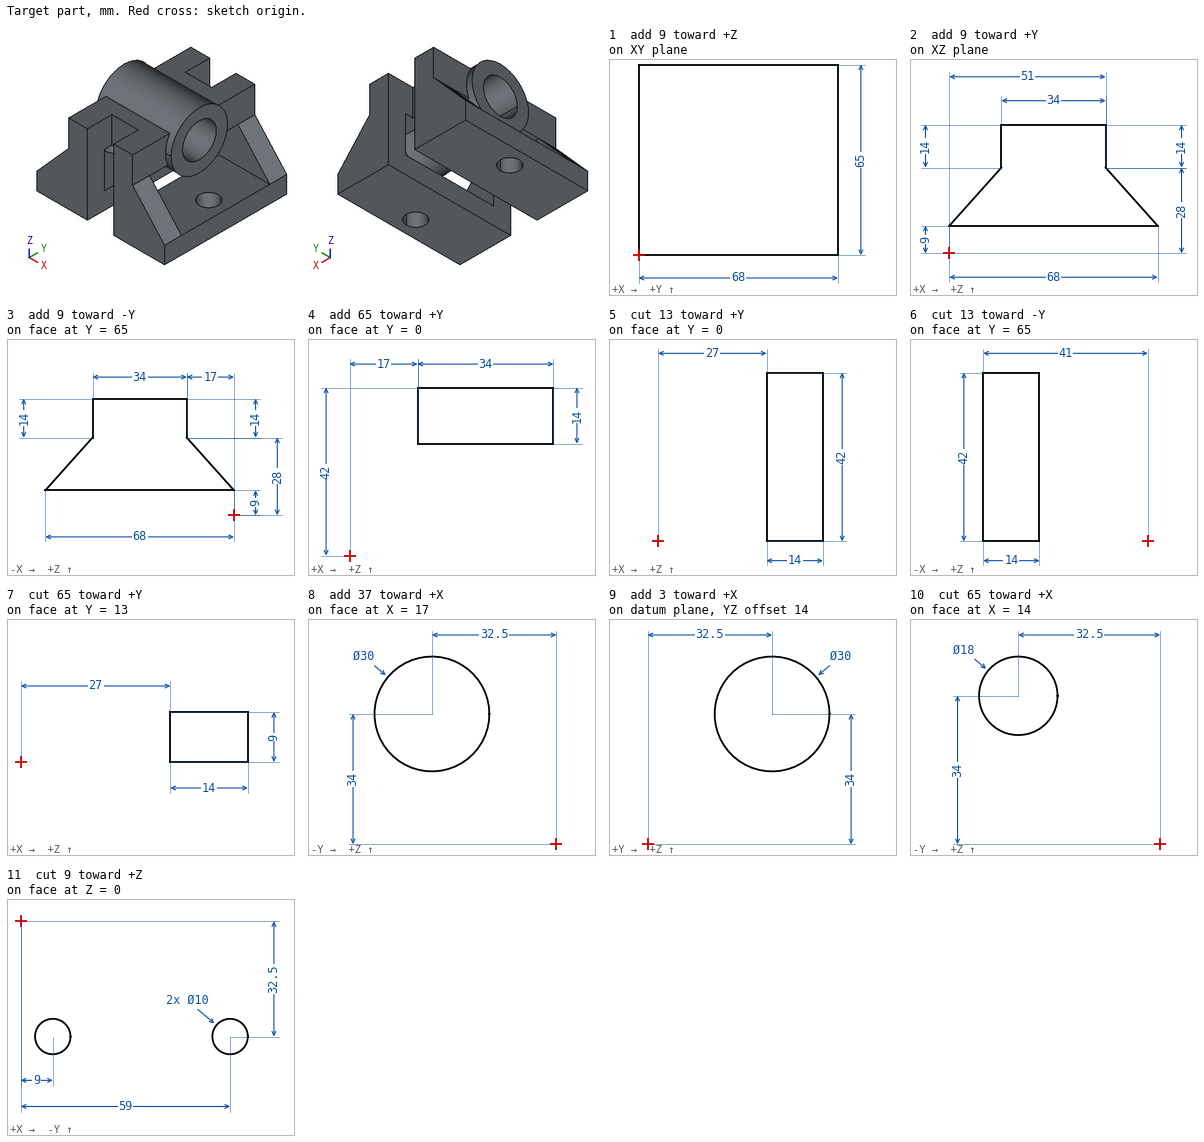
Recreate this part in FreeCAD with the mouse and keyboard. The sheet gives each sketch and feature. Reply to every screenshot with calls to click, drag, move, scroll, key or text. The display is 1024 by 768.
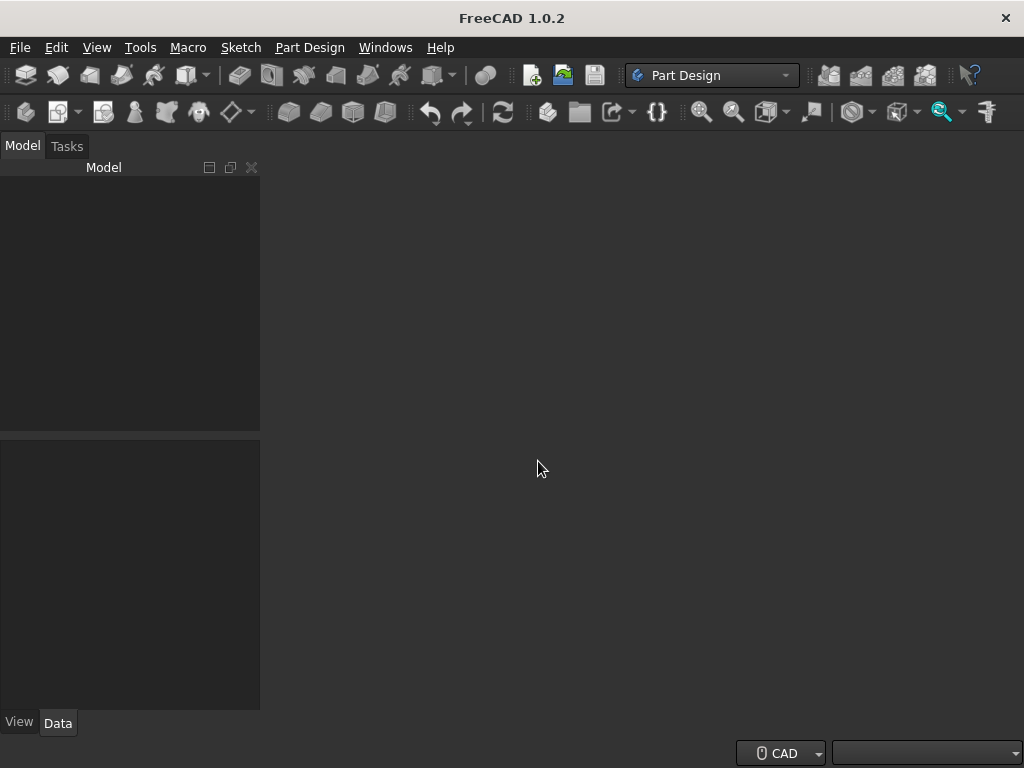
click(532, 76)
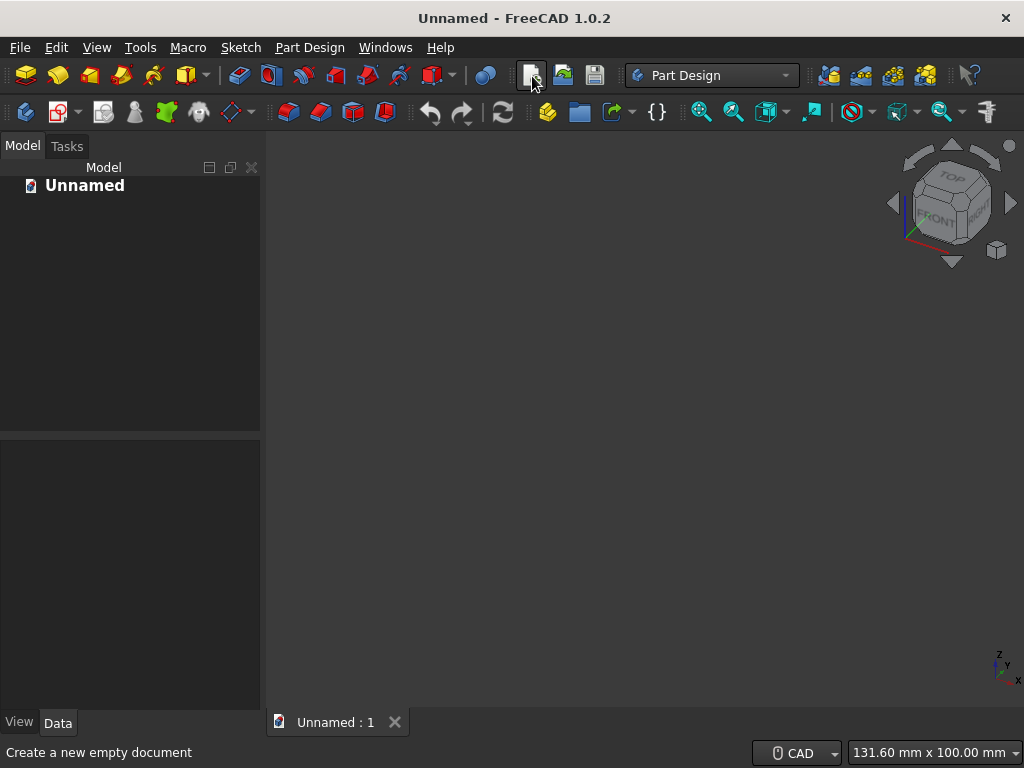
click(58, 112)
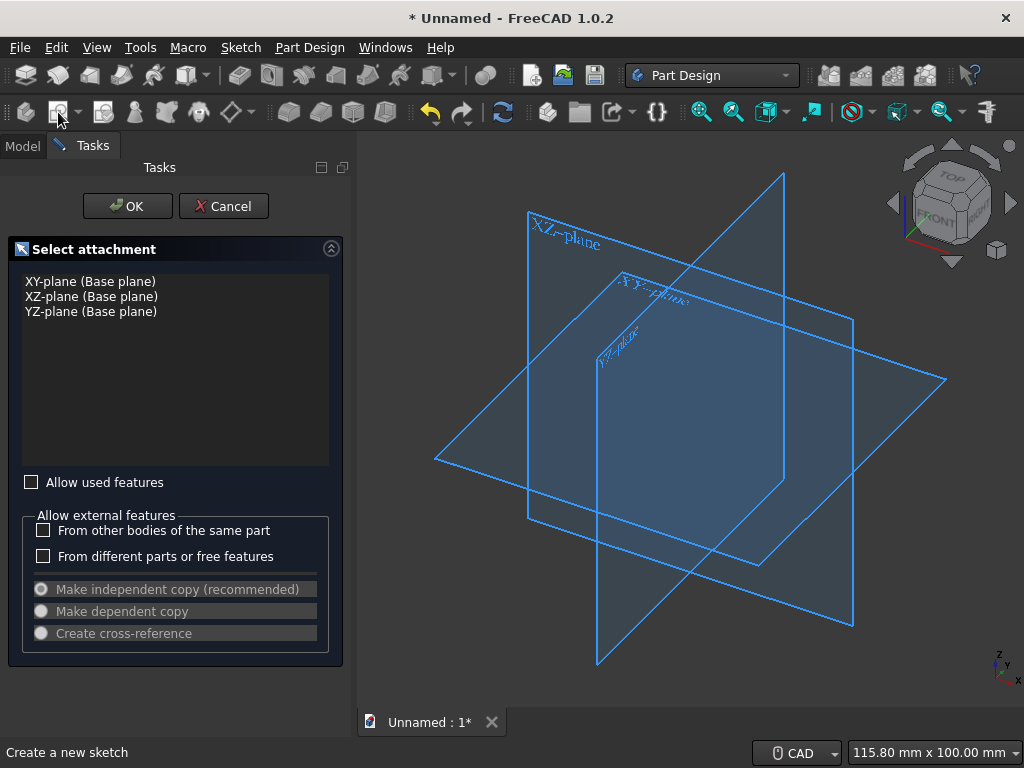
click(82, 282)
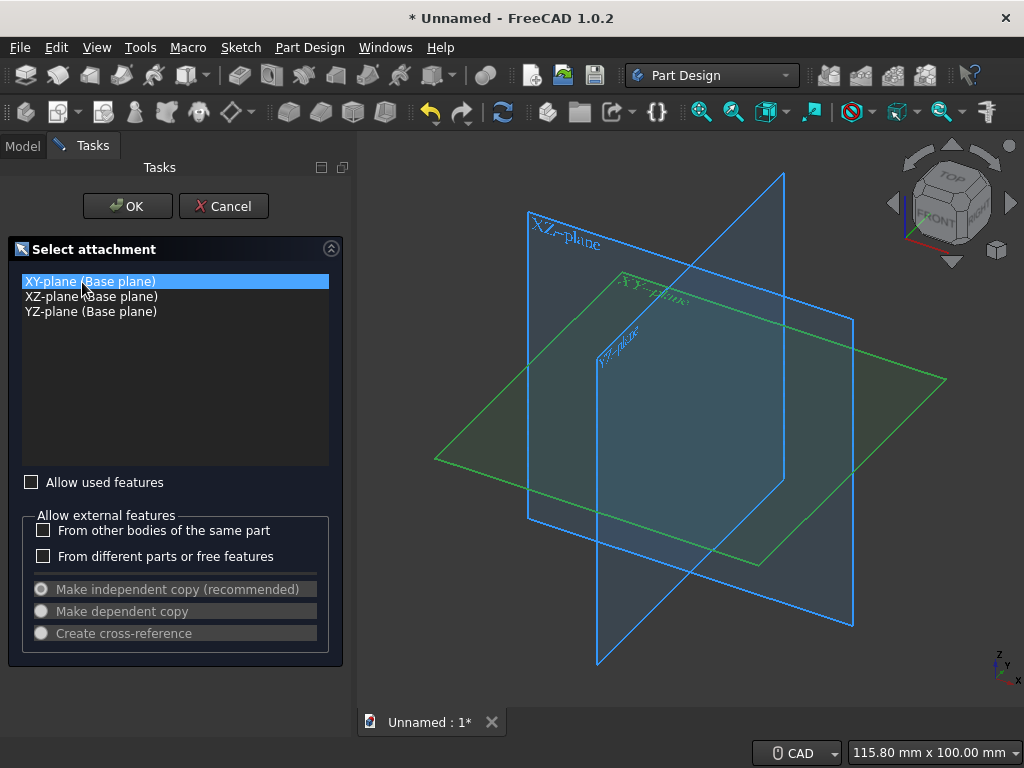
click(128, 206)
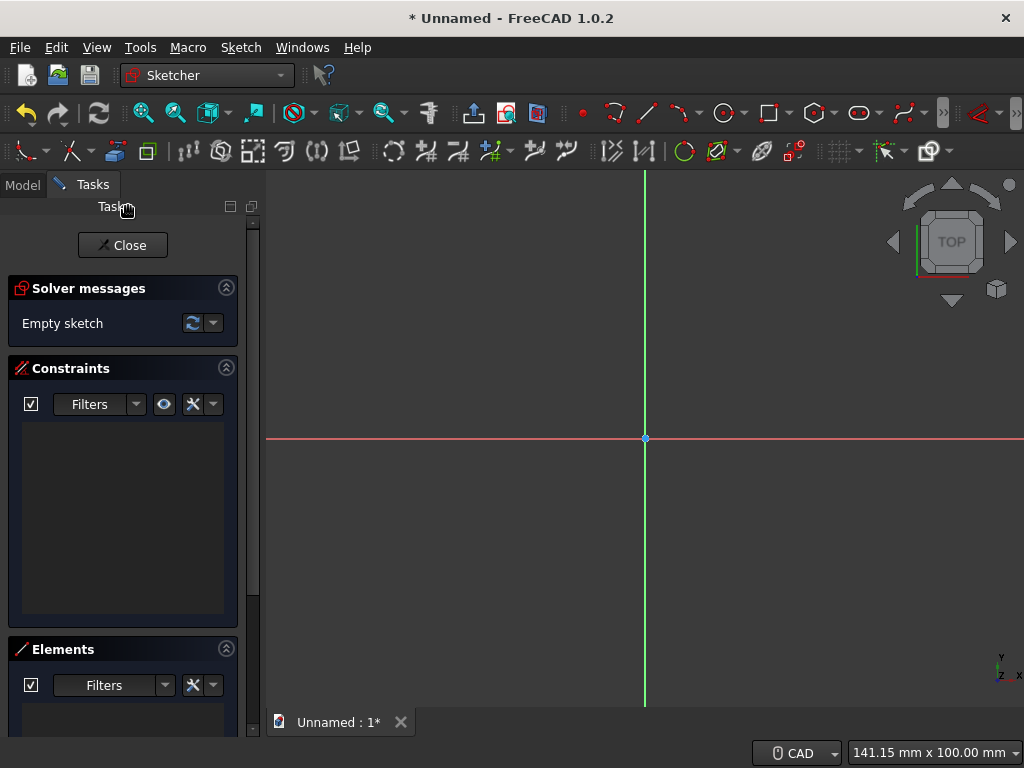
scroll(294, 679, down, 2)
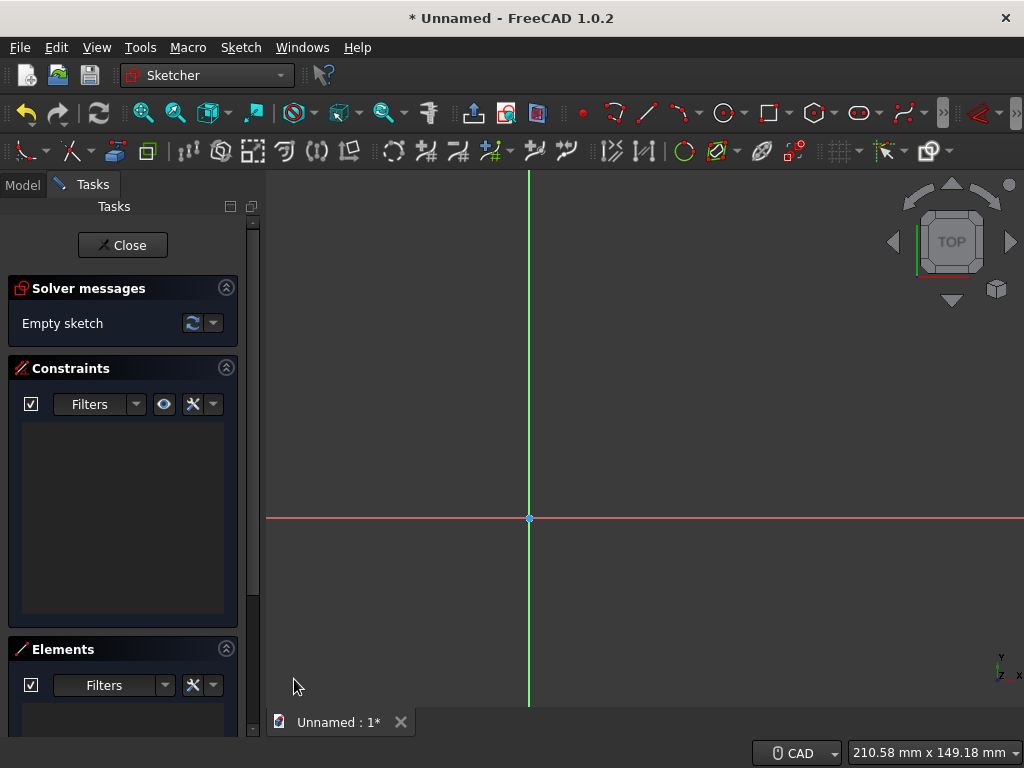
scroll(805, 325, up, 2)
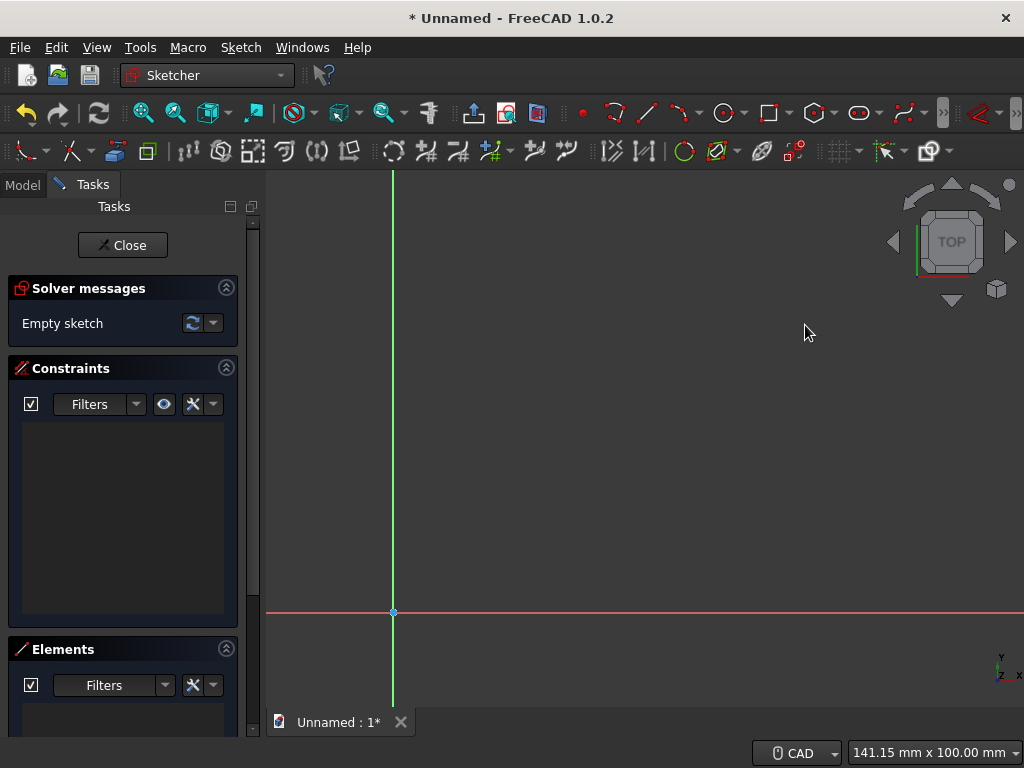
key(g)
key(r)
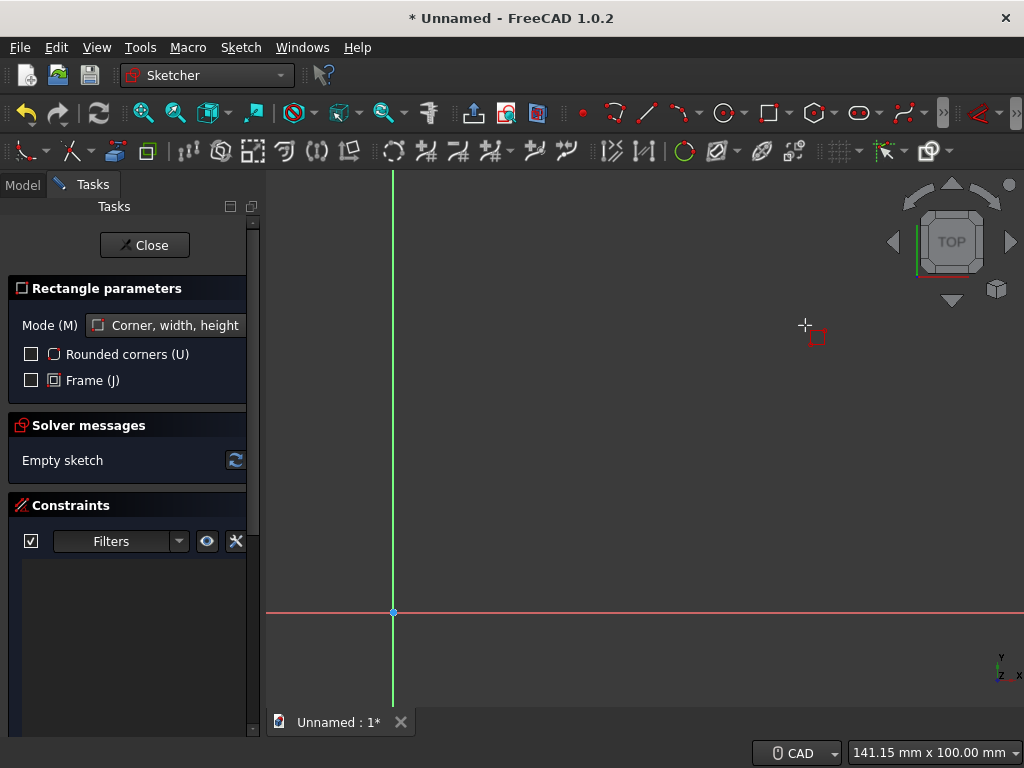
click(393, 613)
move(759, 264)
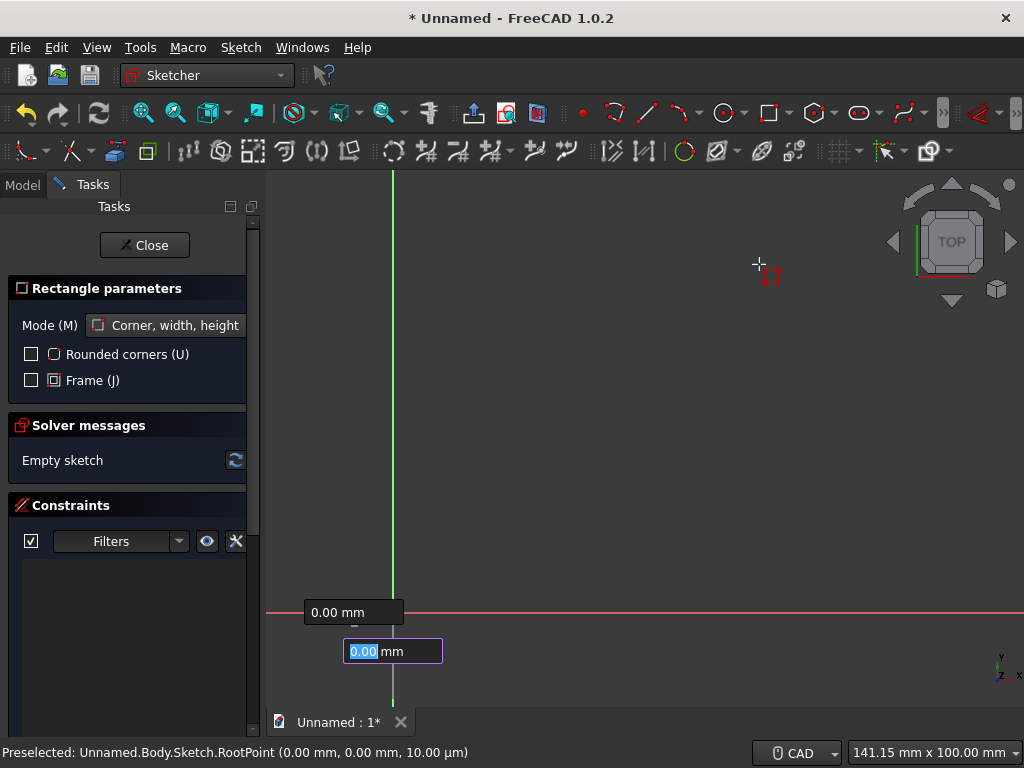
text(68)
key(Tab)
text(65)
key(Return)
key(Escape)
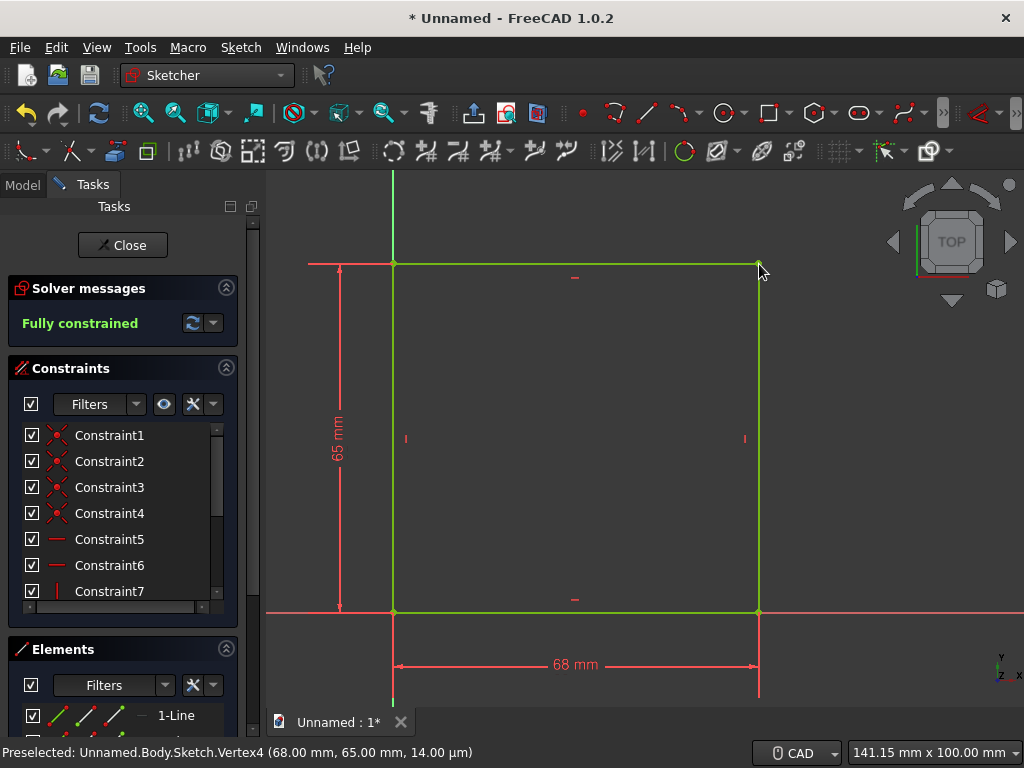
click(123, 245)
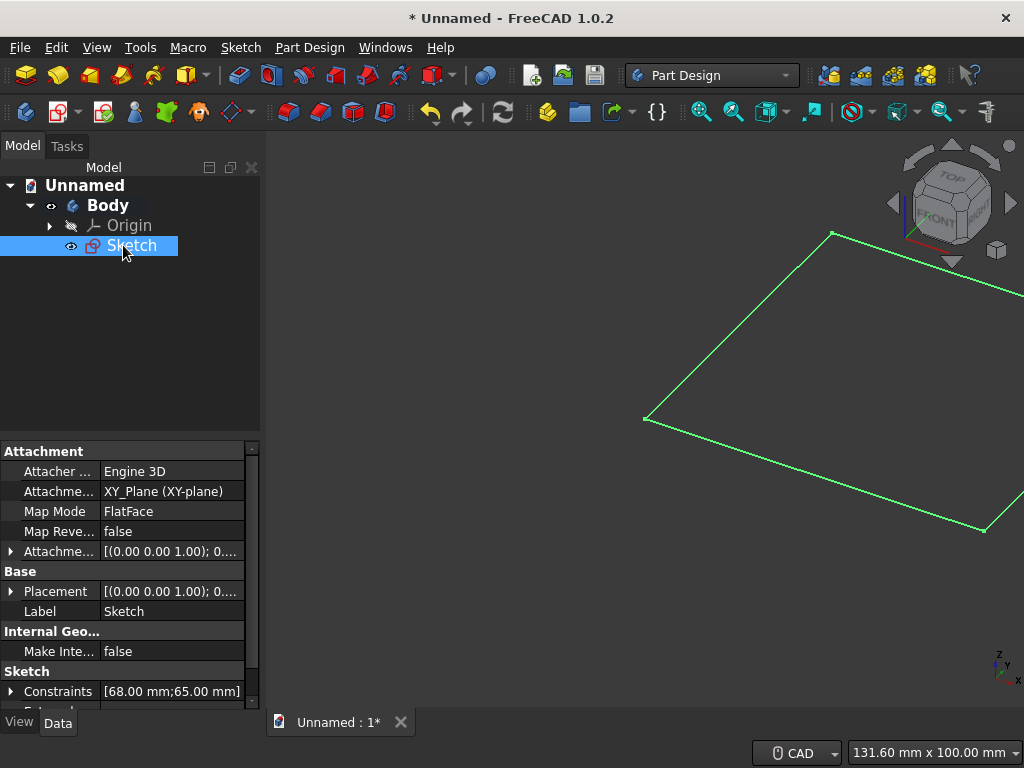
click(26, 76)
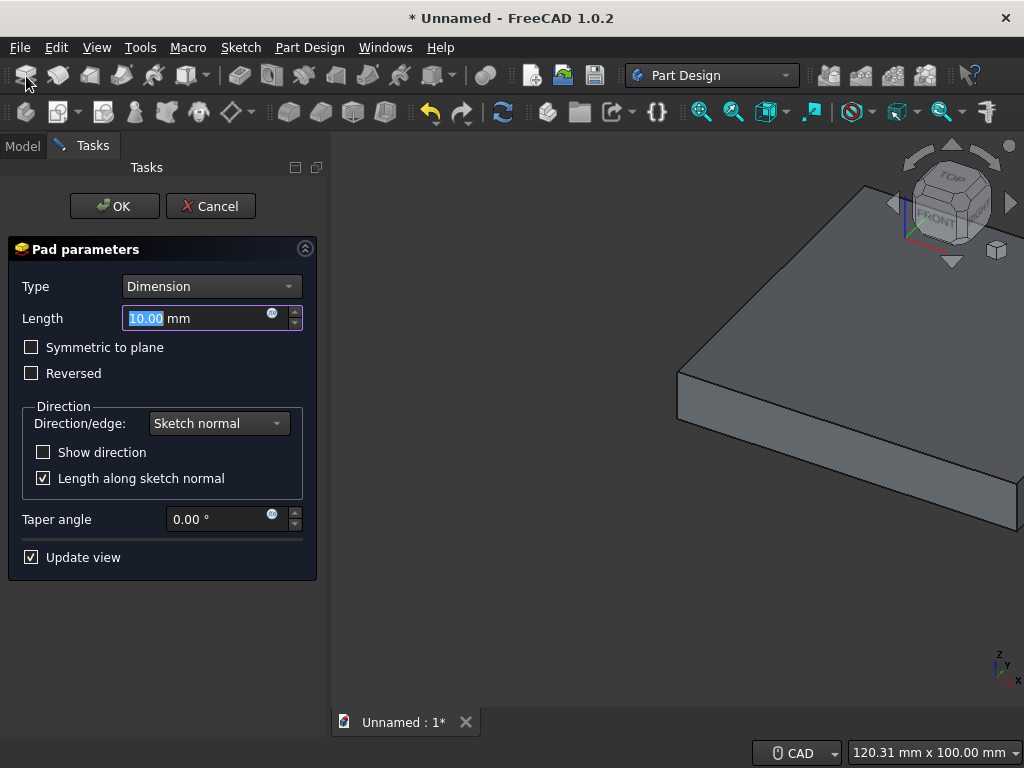
text(9)
key(Tab)